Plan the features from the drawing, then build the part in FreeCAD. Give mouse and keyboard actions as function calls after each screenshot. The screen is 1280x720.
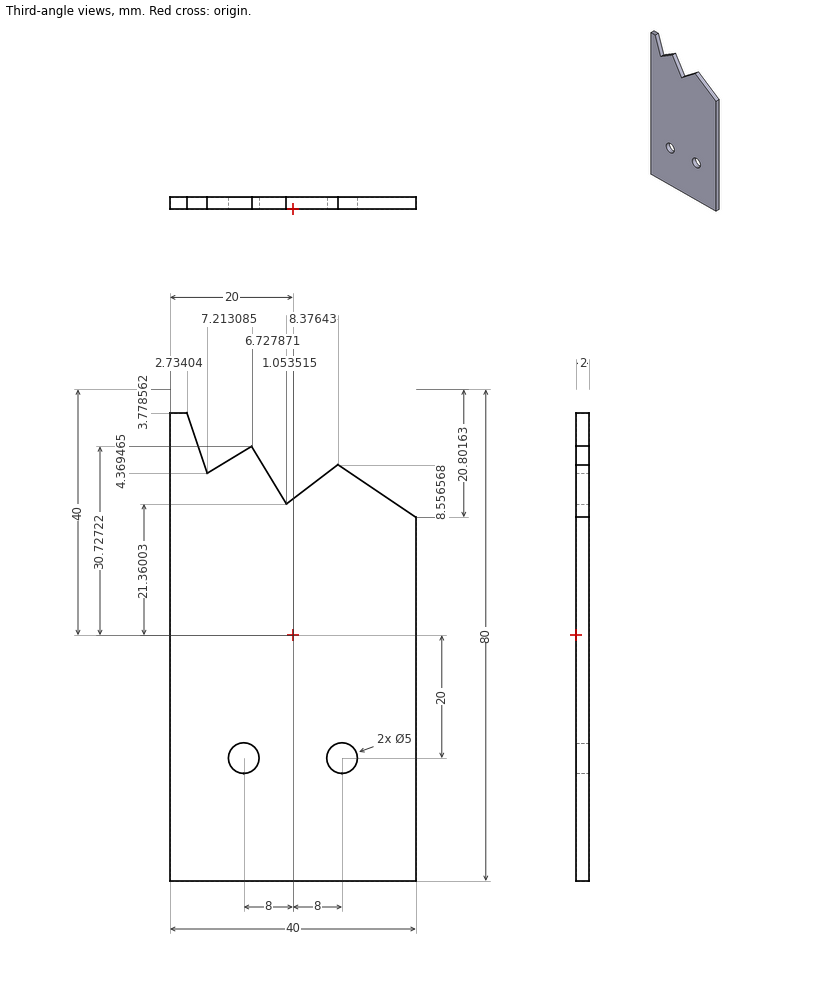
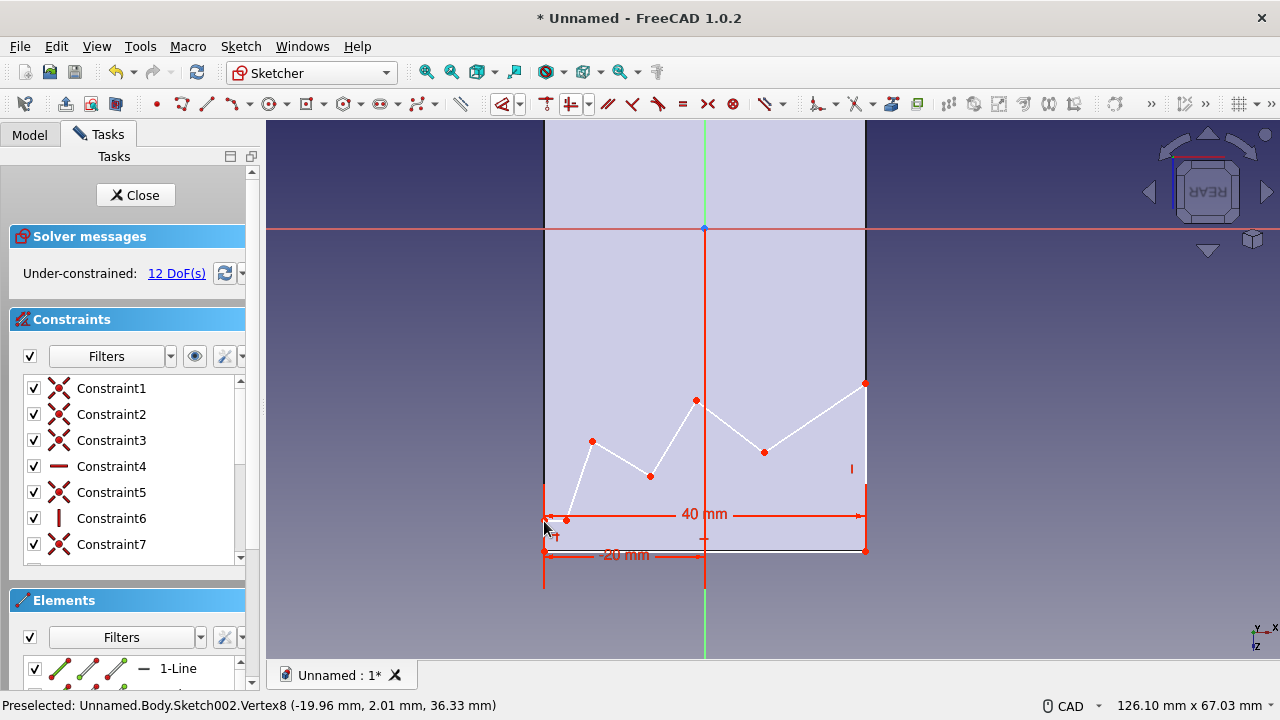
click(544, 552)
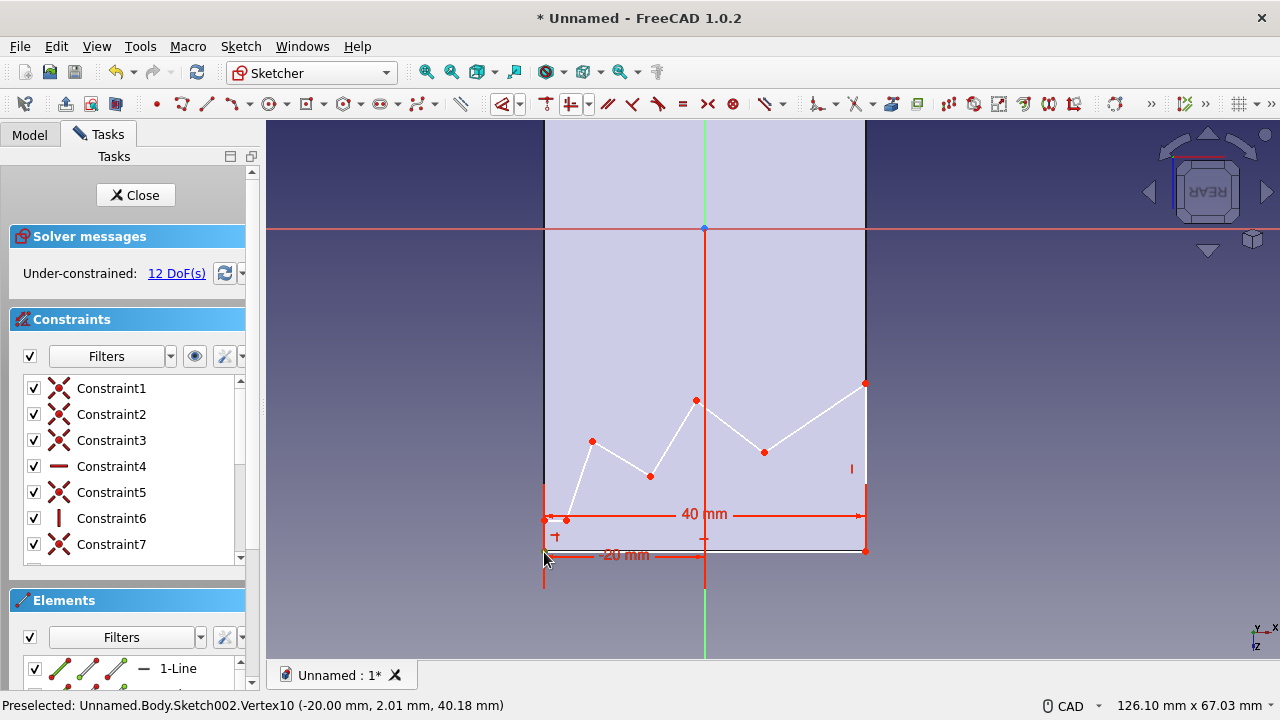
key(i)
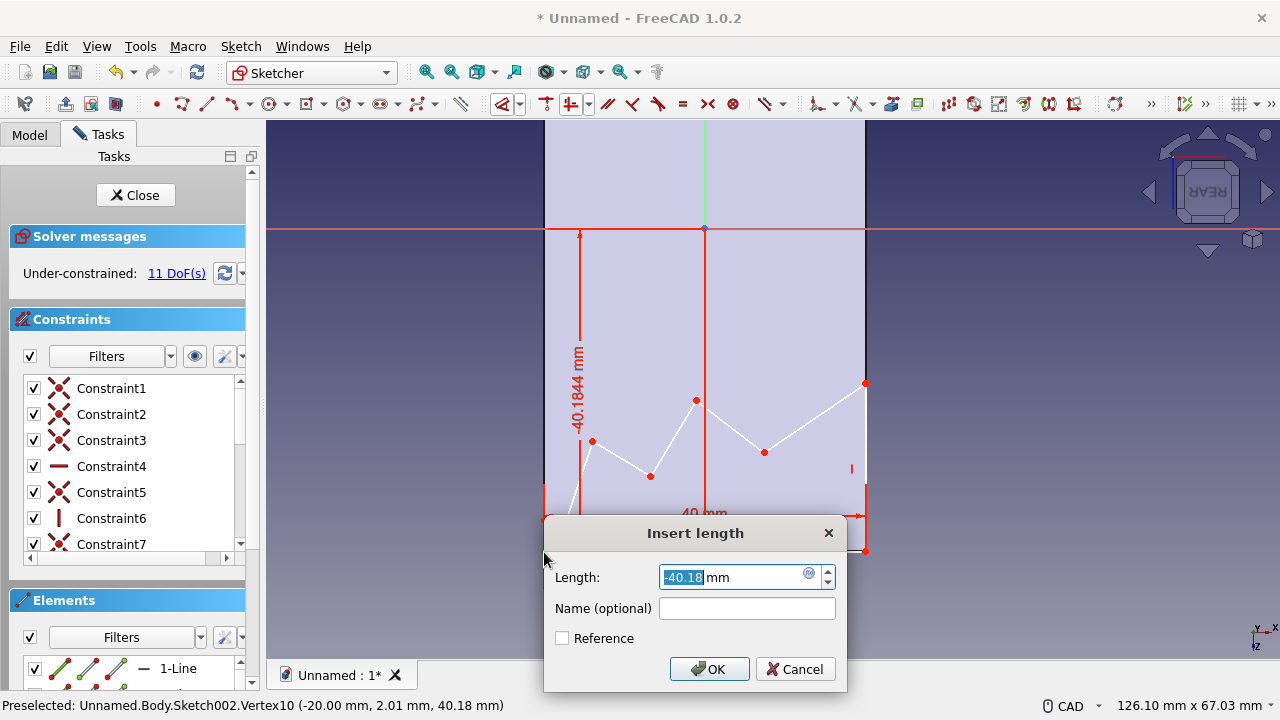
text(-40)
key(Return)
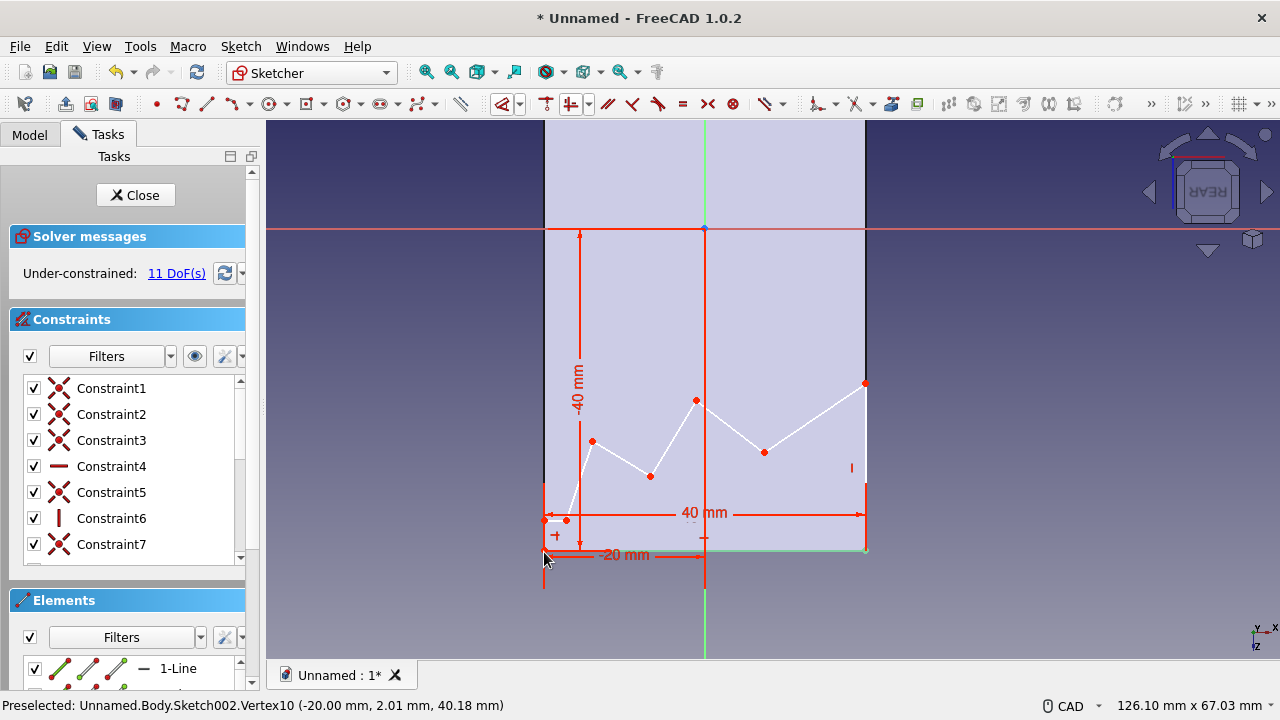
scroll(555, 521, up, 3)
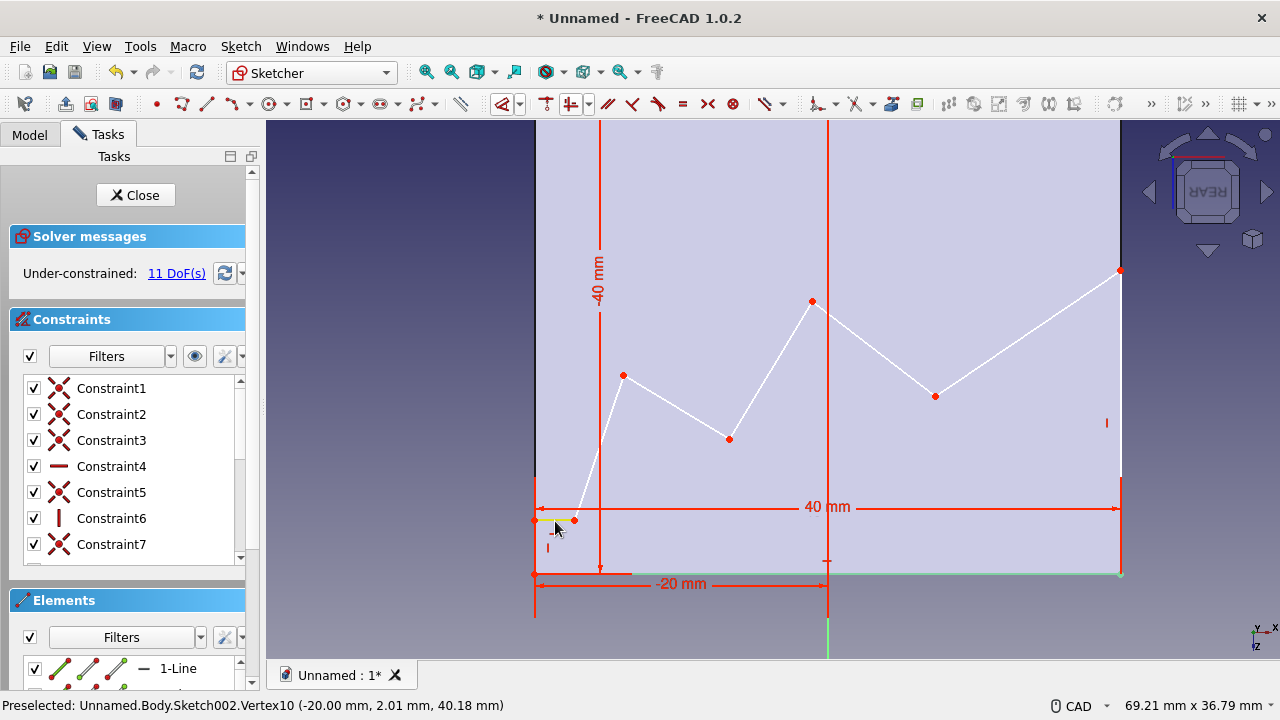
click(555, 520)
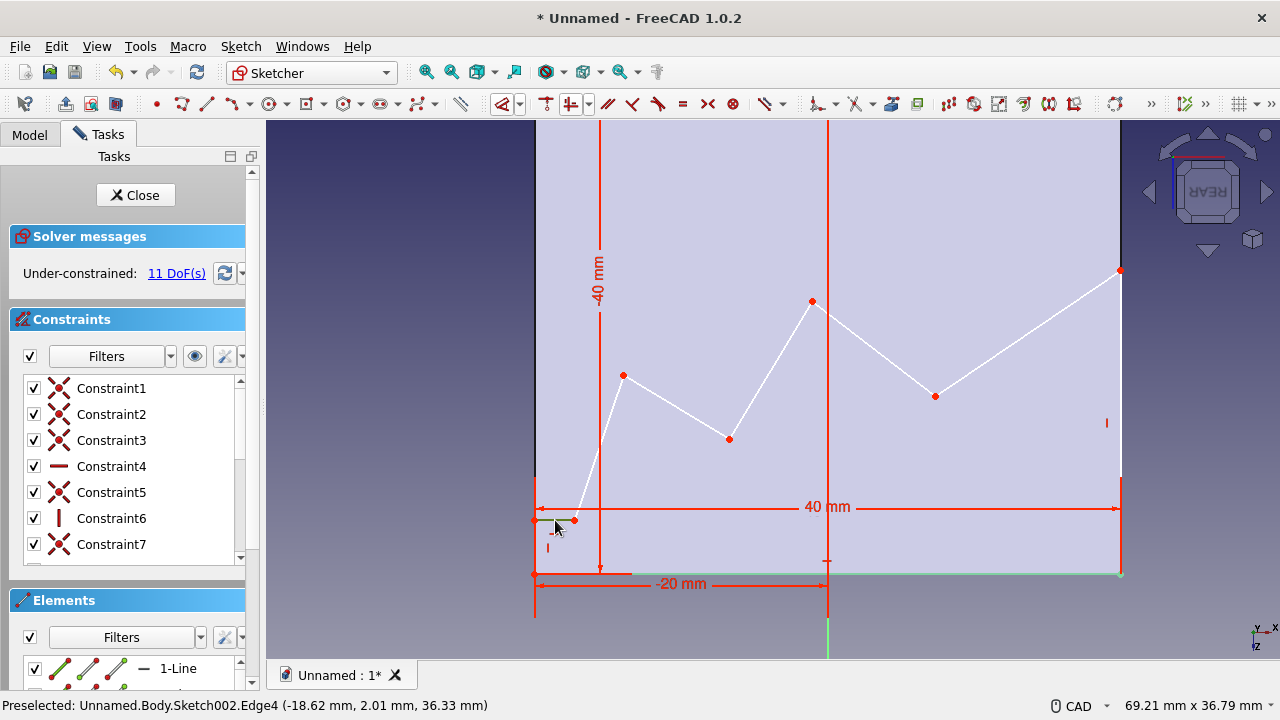
key(l)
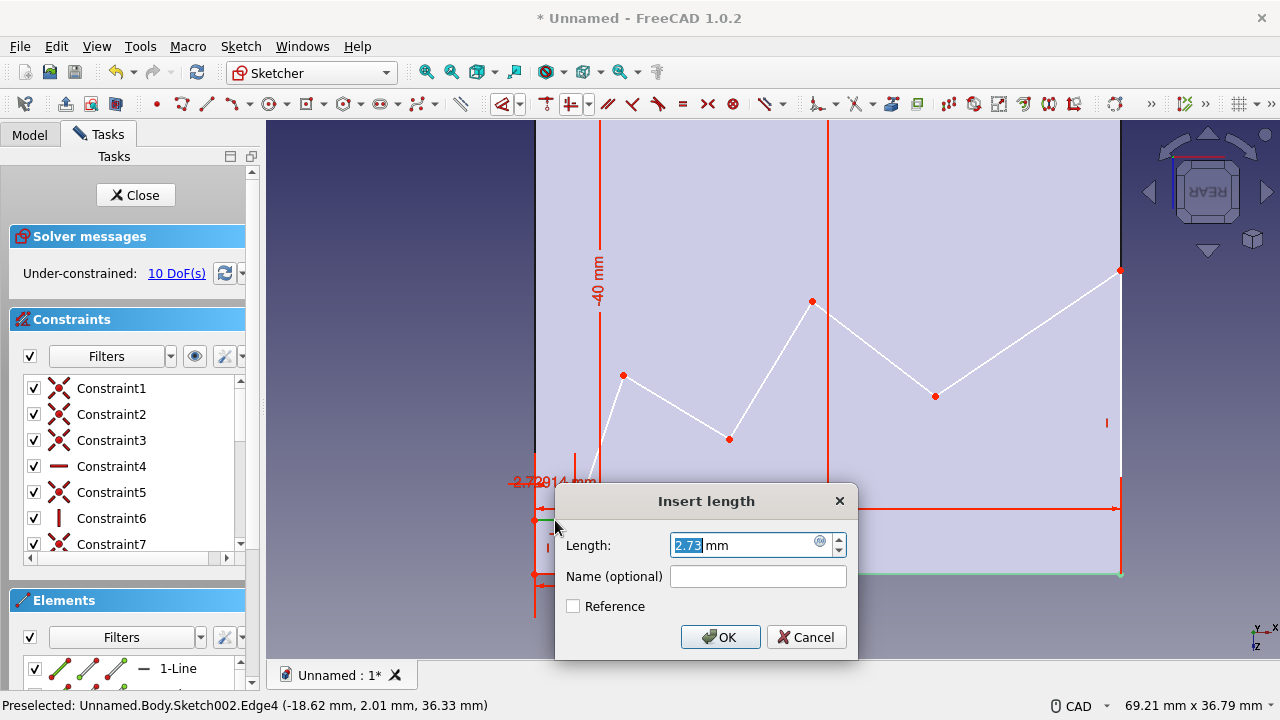
text(2.73404)
key(Return)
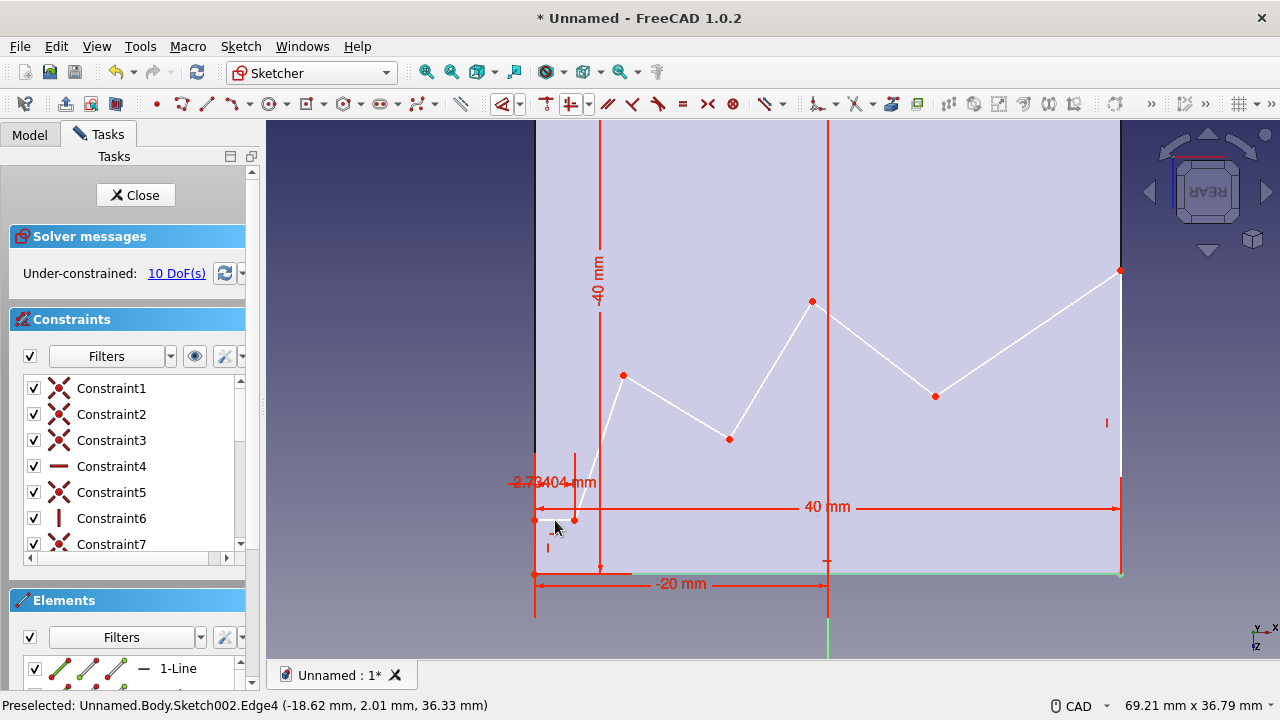
click(535, 537)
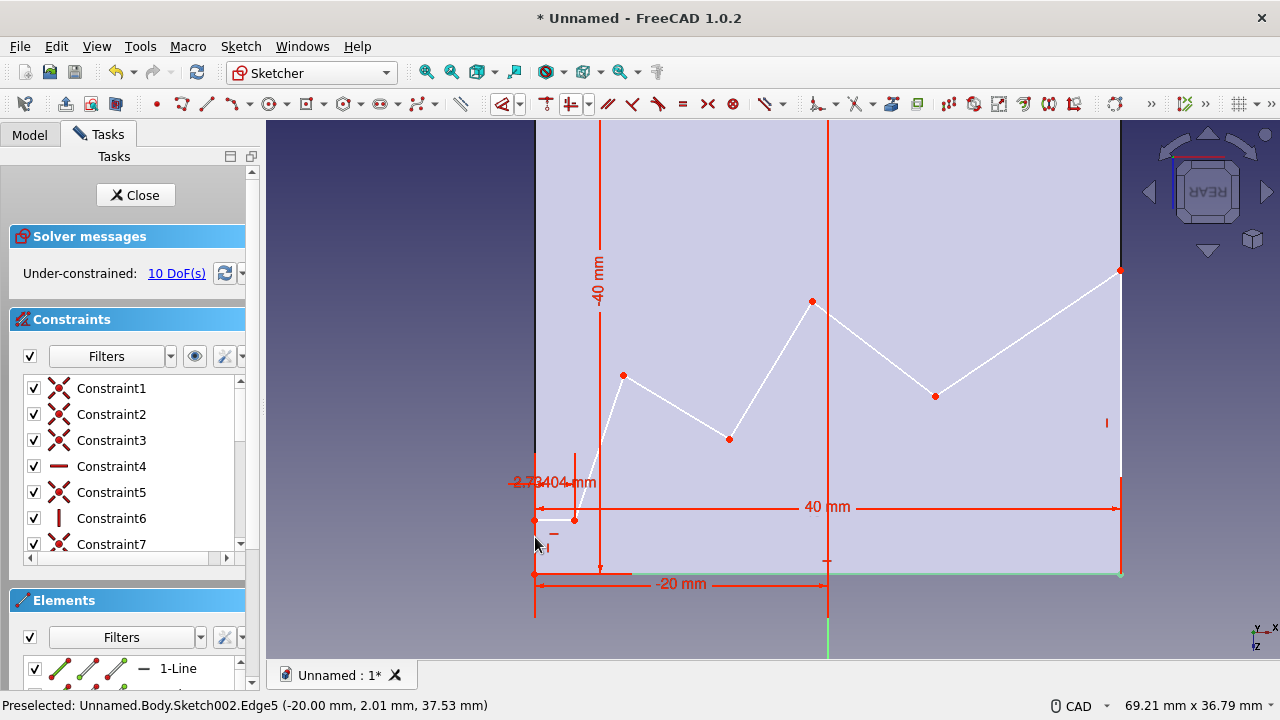
key(i)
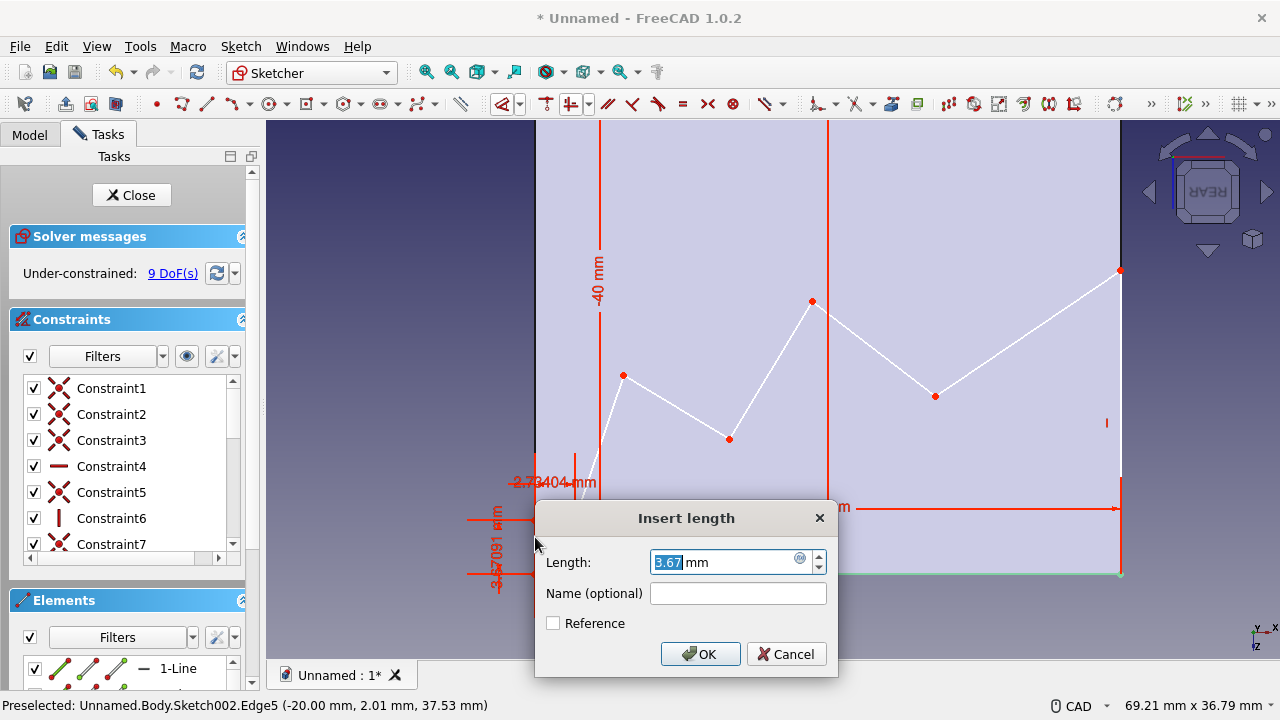
text(3.778562)
key(Return)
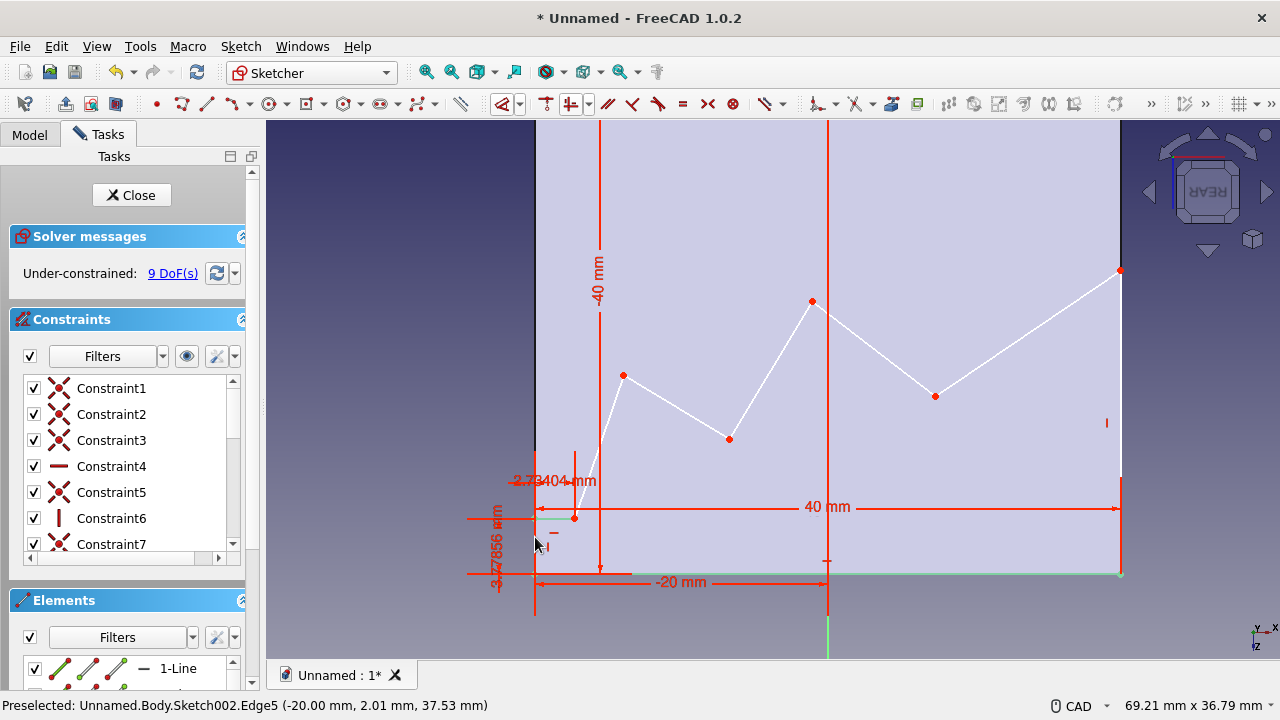
scroll(554, 521, down, 3)